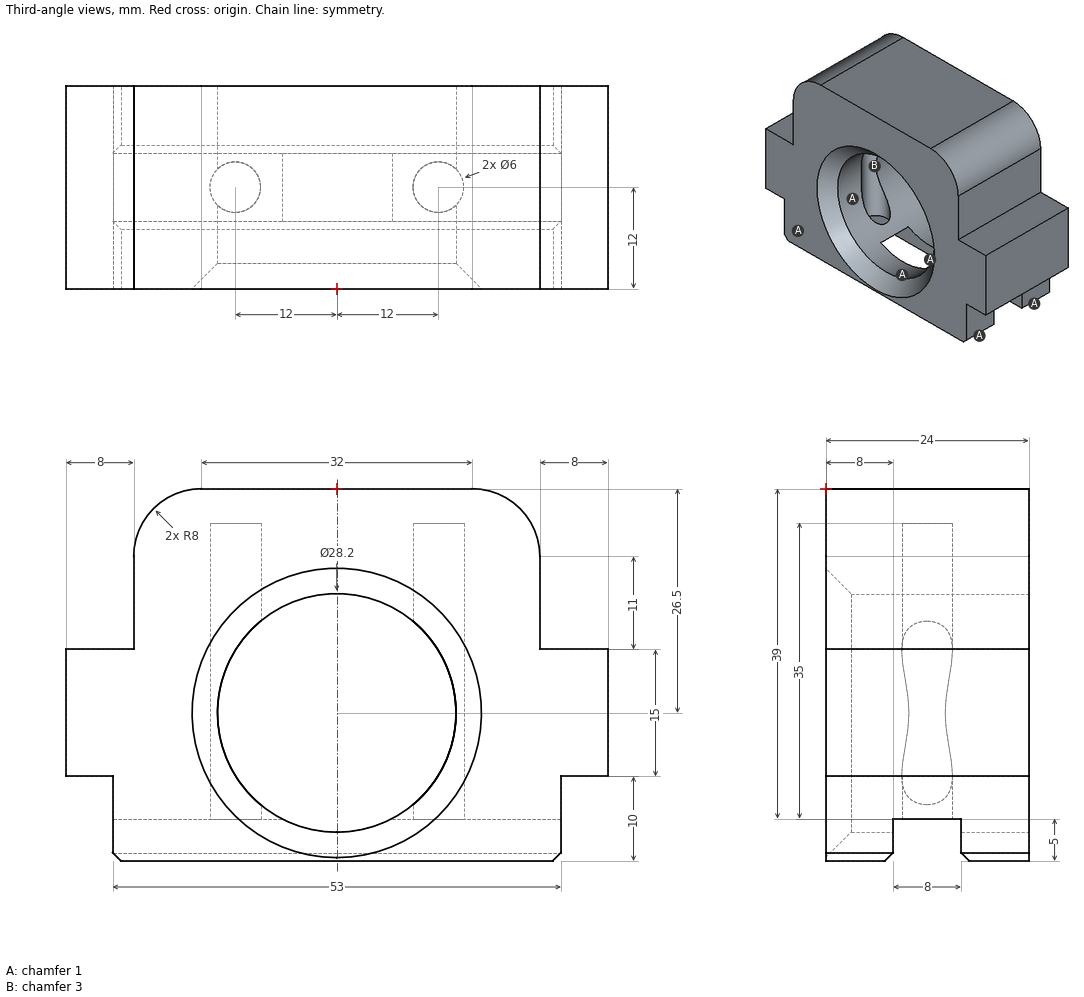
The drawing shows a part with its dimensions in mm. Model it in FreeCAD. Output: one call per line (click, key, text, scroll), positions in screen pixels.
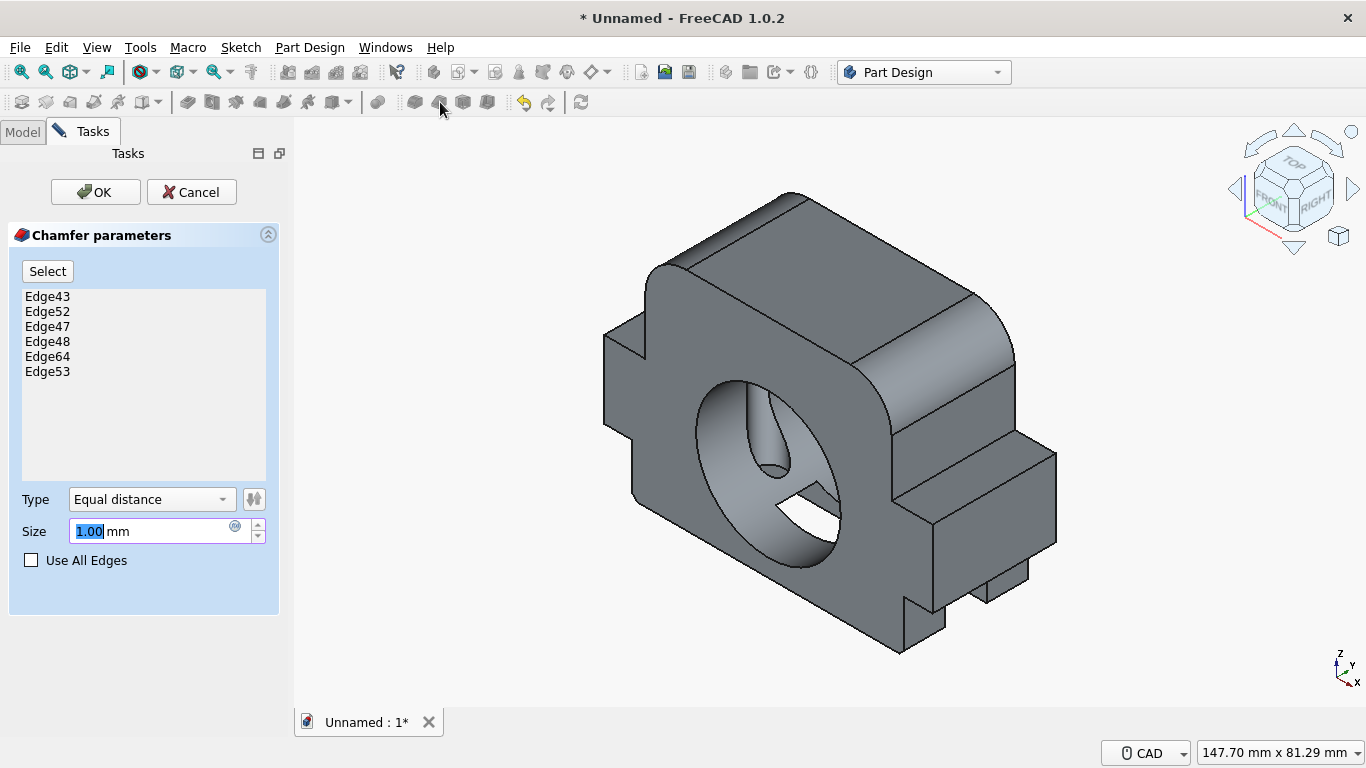
text(1)
key(Tab)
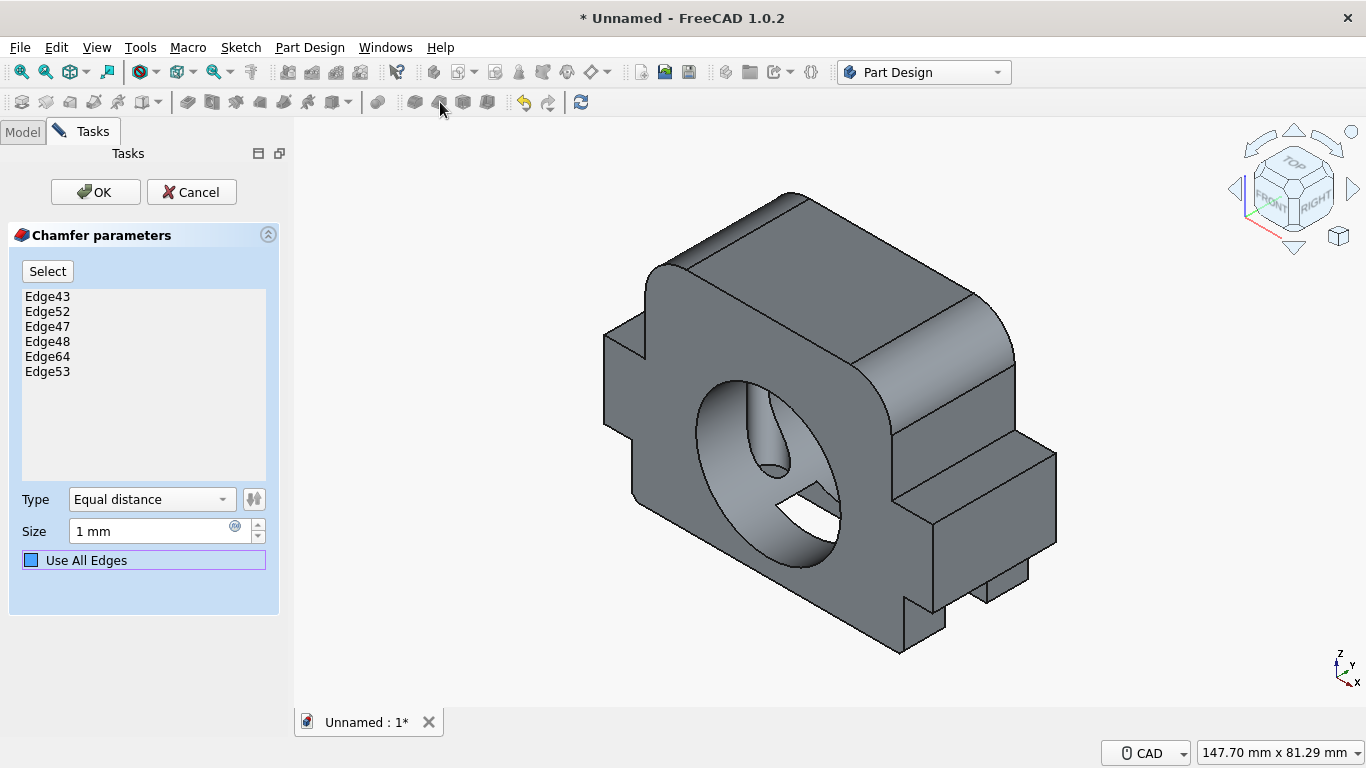
click(96, 192)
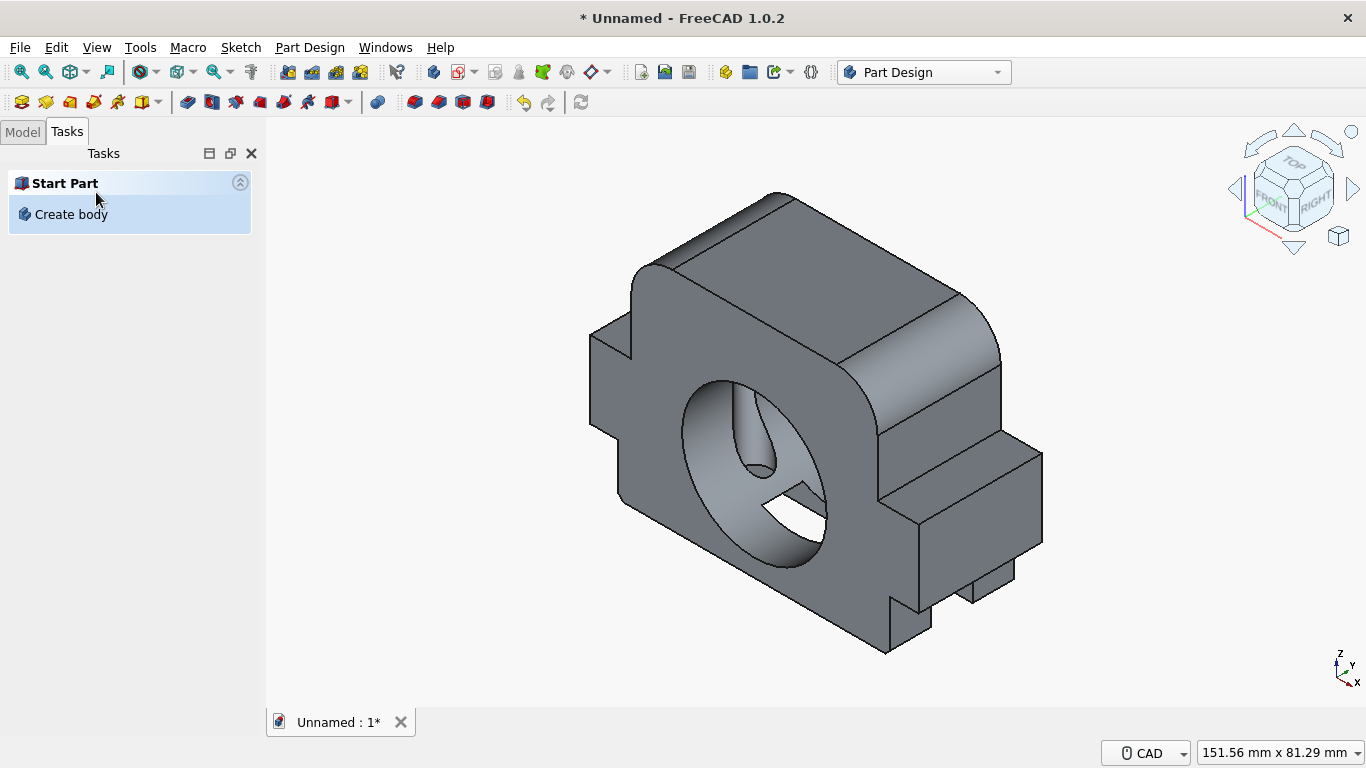
click(682, 431)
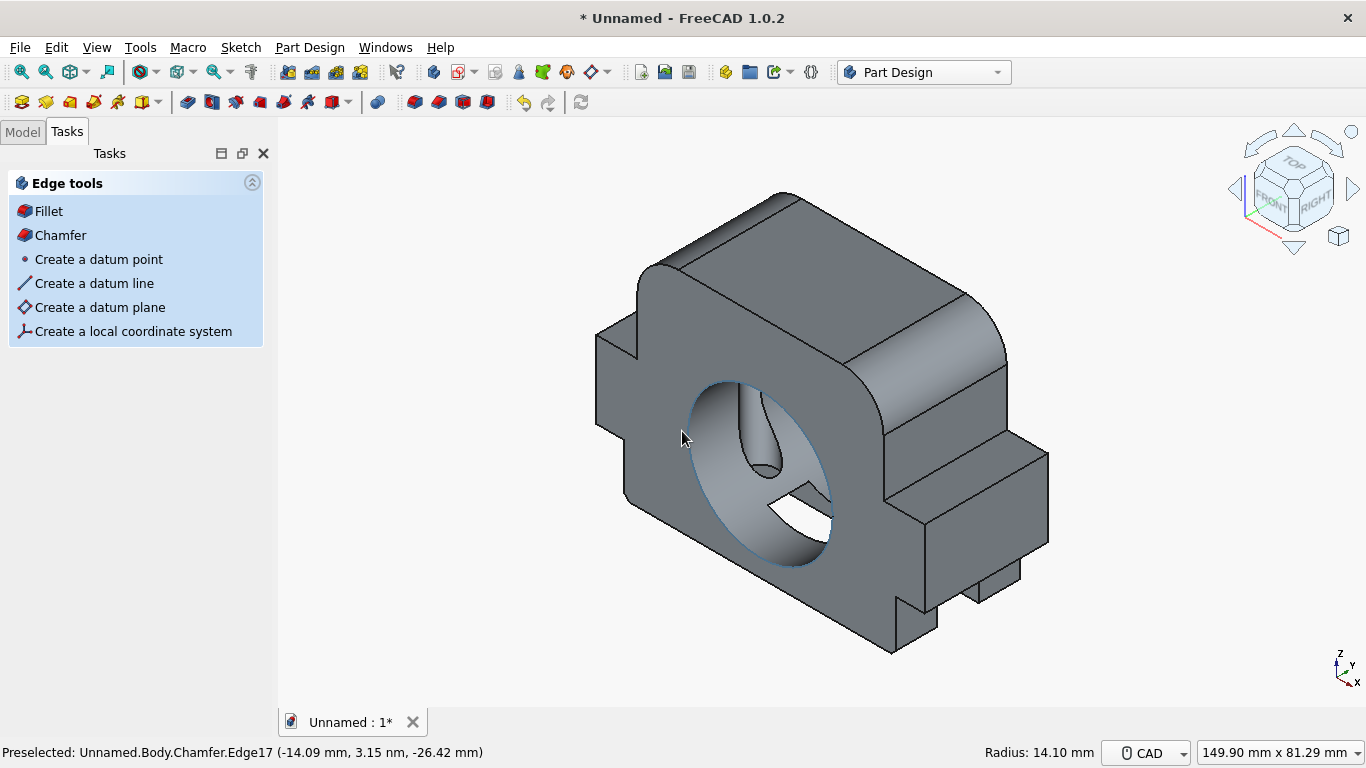
click(440, 102)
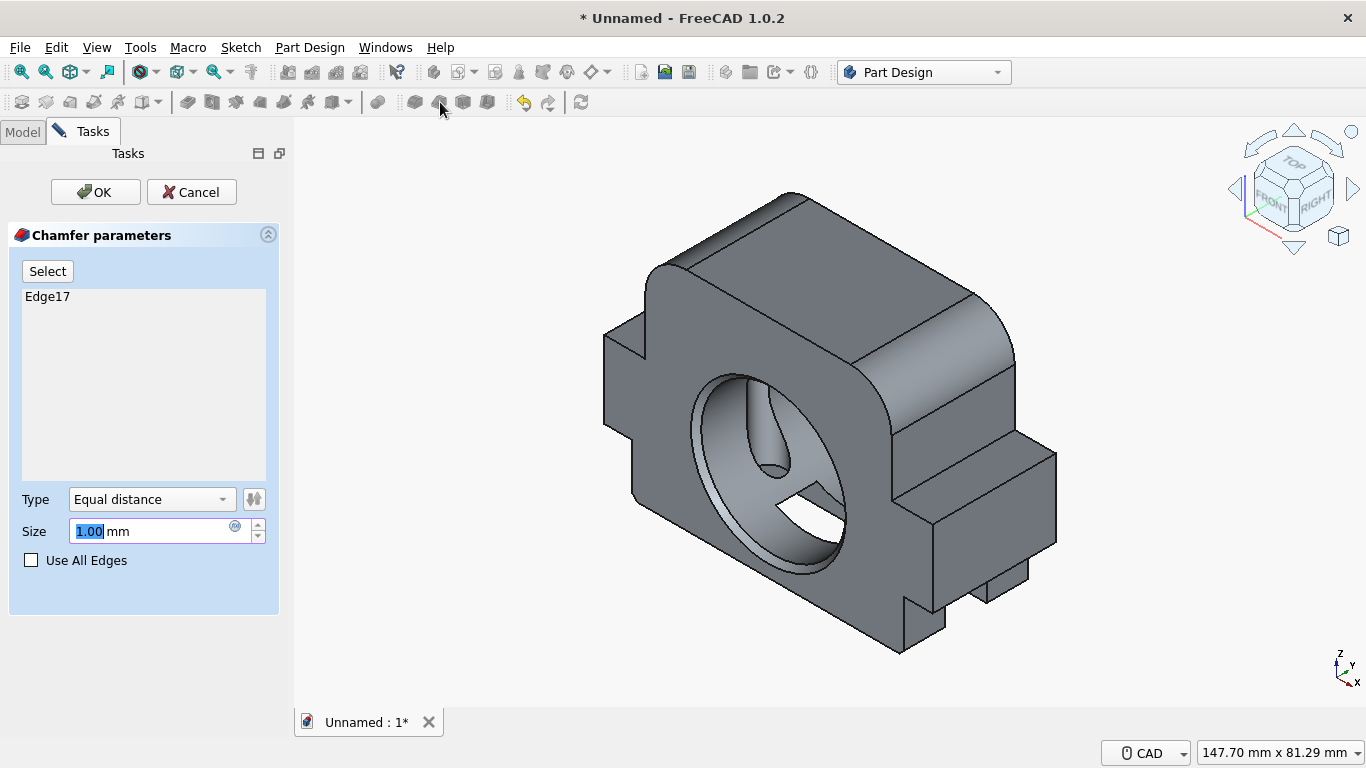
text(3)
key(Tab)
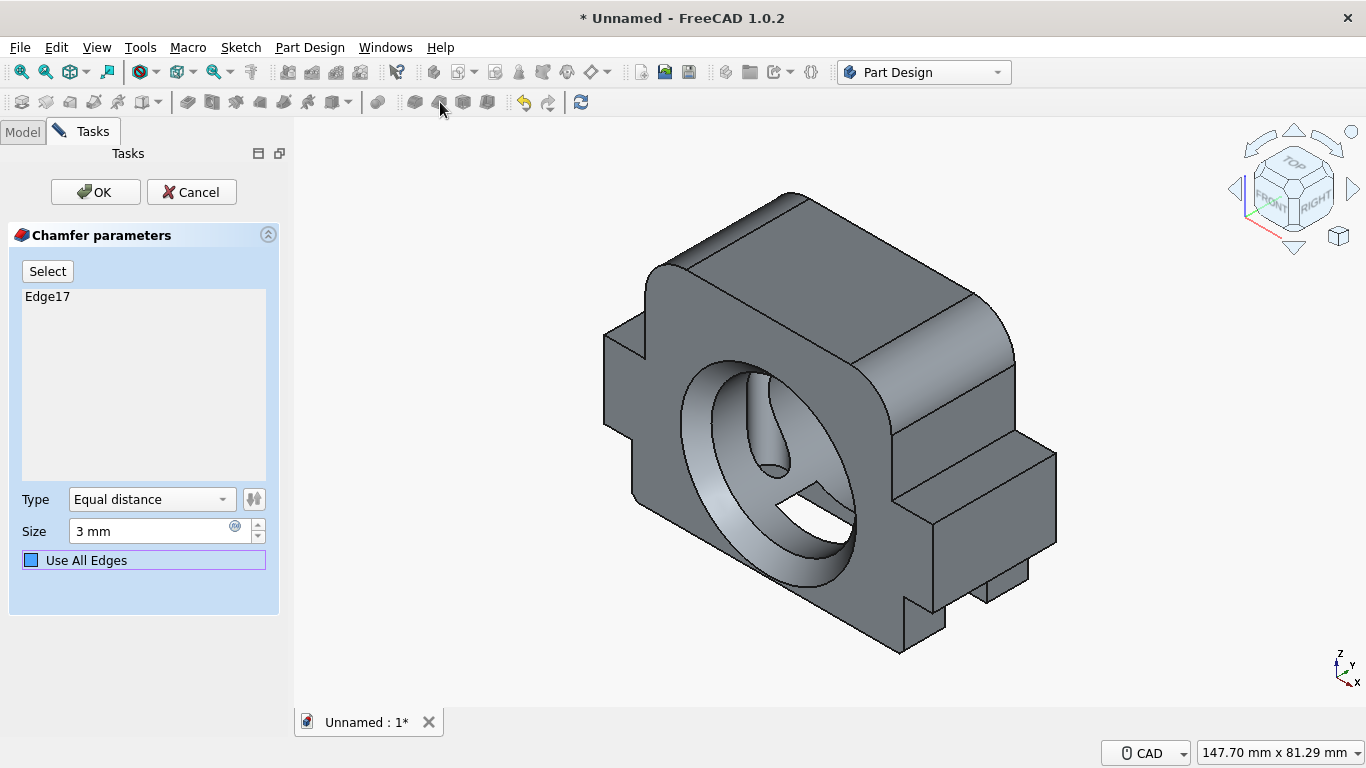
click(96, 192)